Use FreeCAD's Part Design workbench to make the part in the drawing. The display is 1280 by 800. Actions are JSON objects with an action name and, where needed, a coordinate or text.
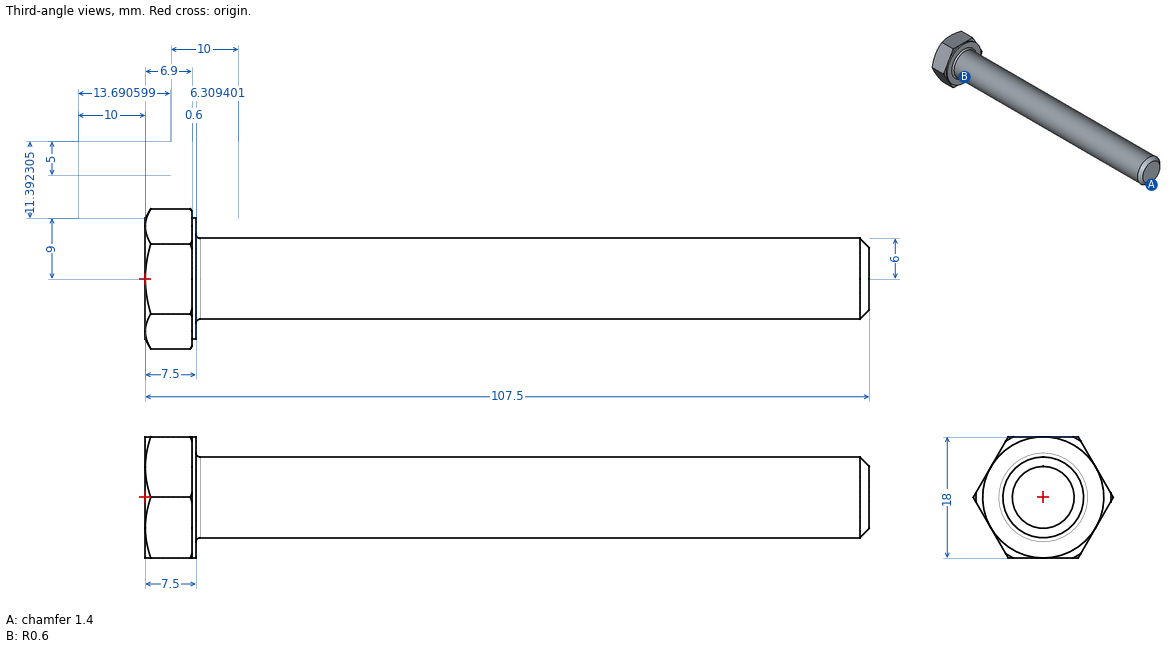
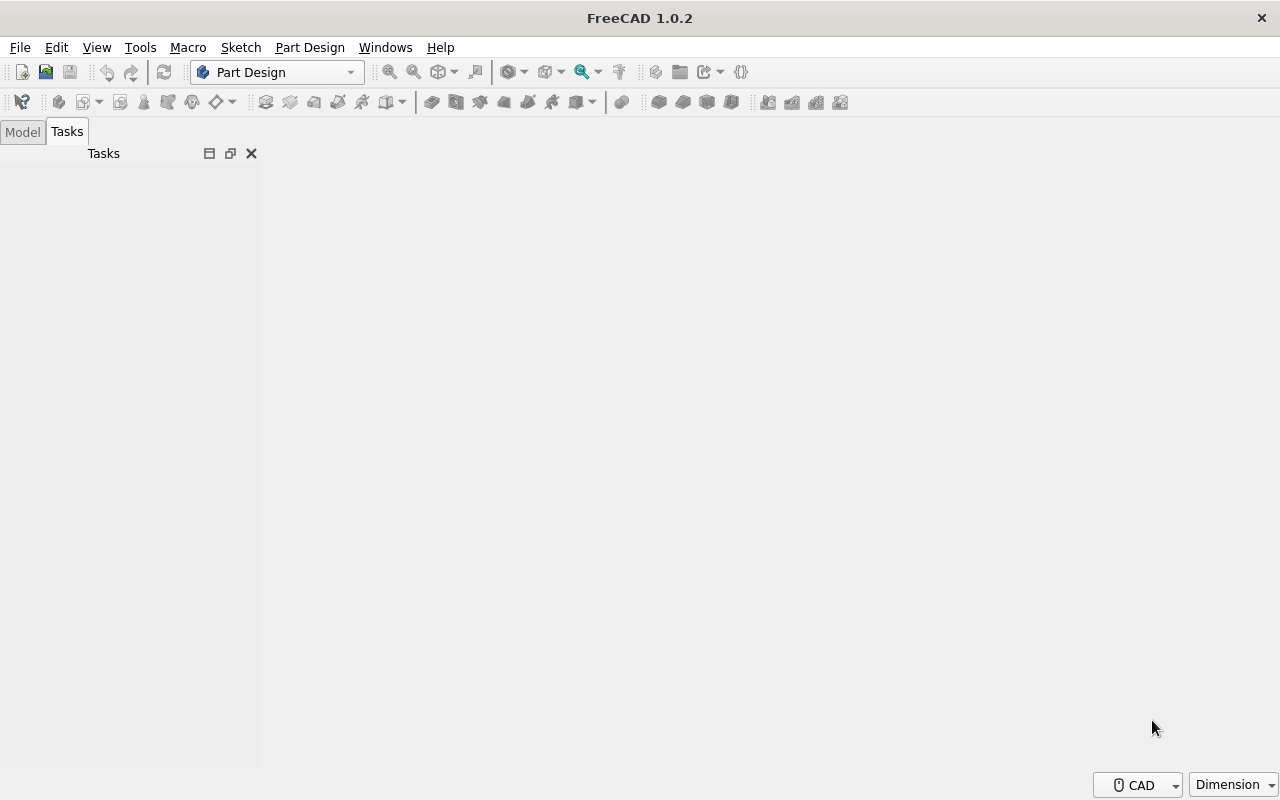
{"action": "key", "text": "ctrl+n"}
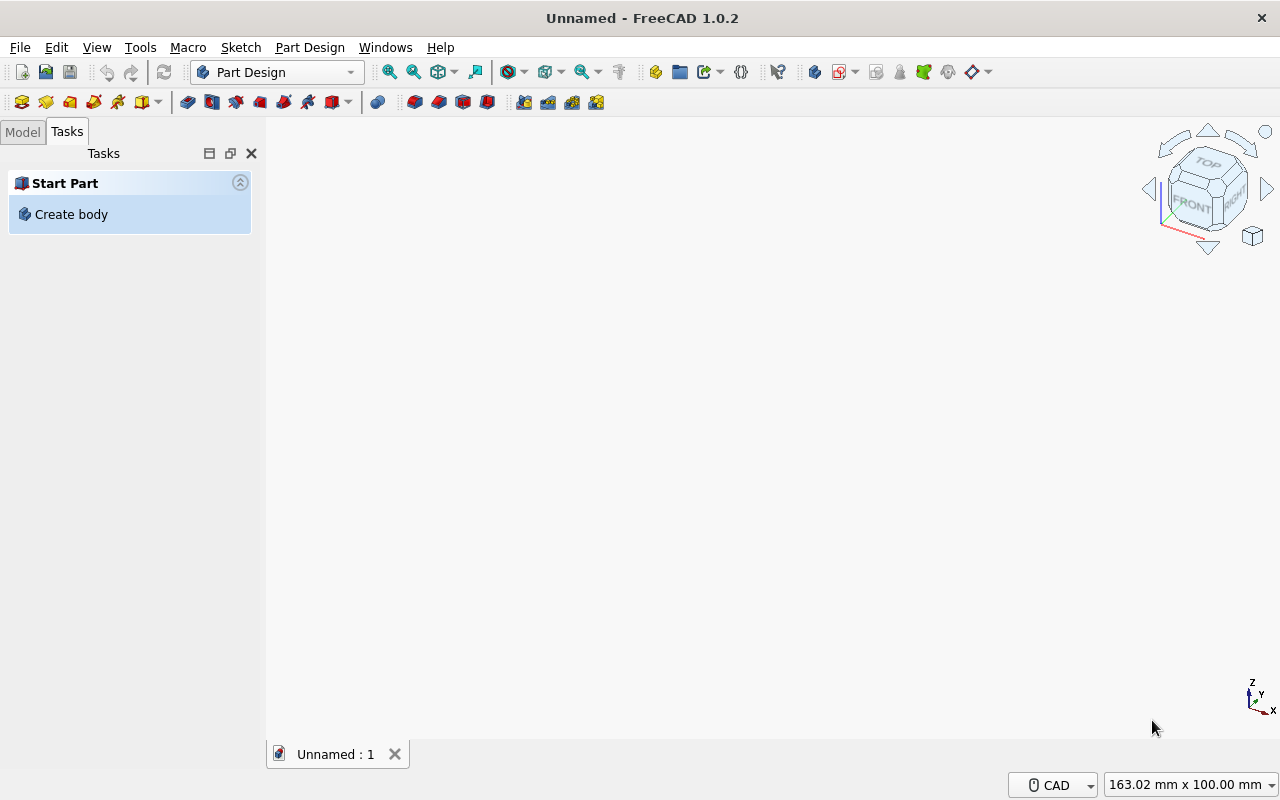
{"action": "left_click", "coordinate": [840, 72]}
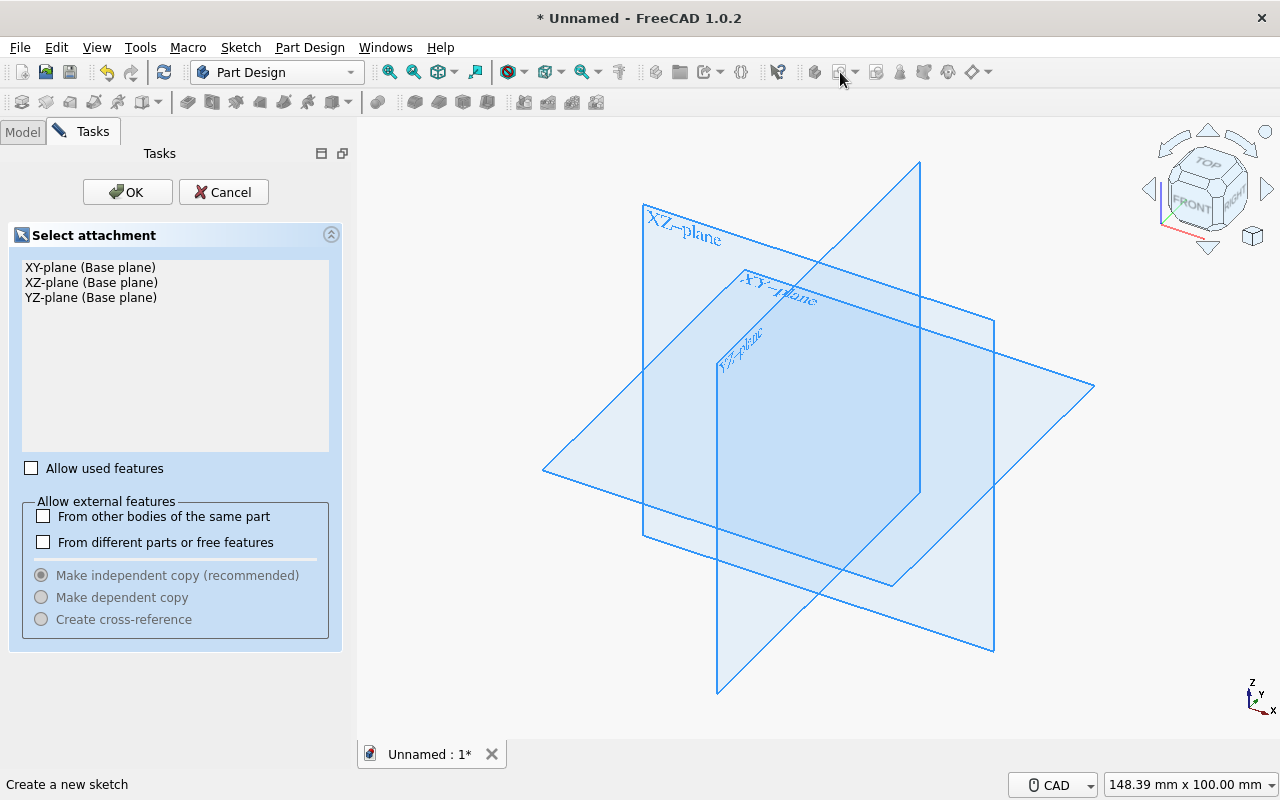
{"action": "left_click", "coordinate": [82, 298]}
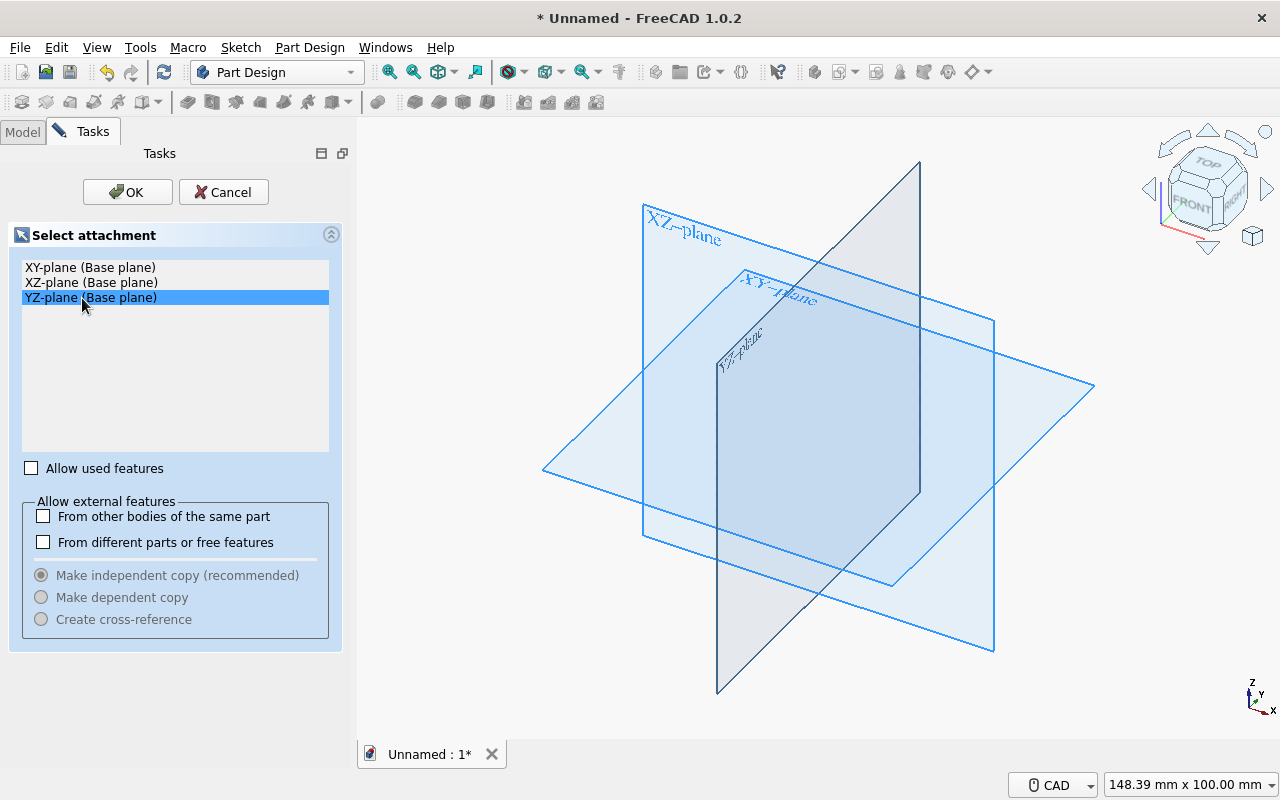
{"action": "left_click", "coordinate": [128, 192]}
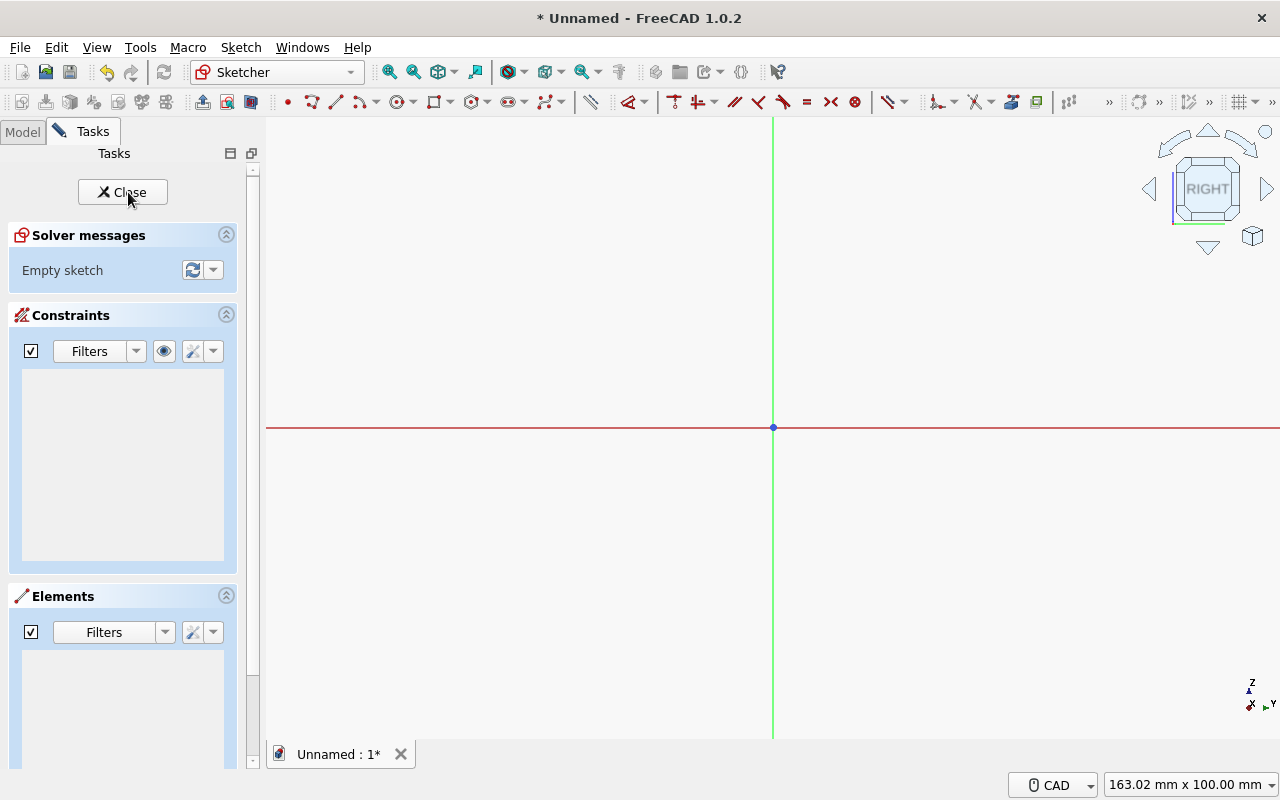
{"action": "scroll", "coordinate": [803, 428], "scroll_direction": "up", "scroll_amount": 6}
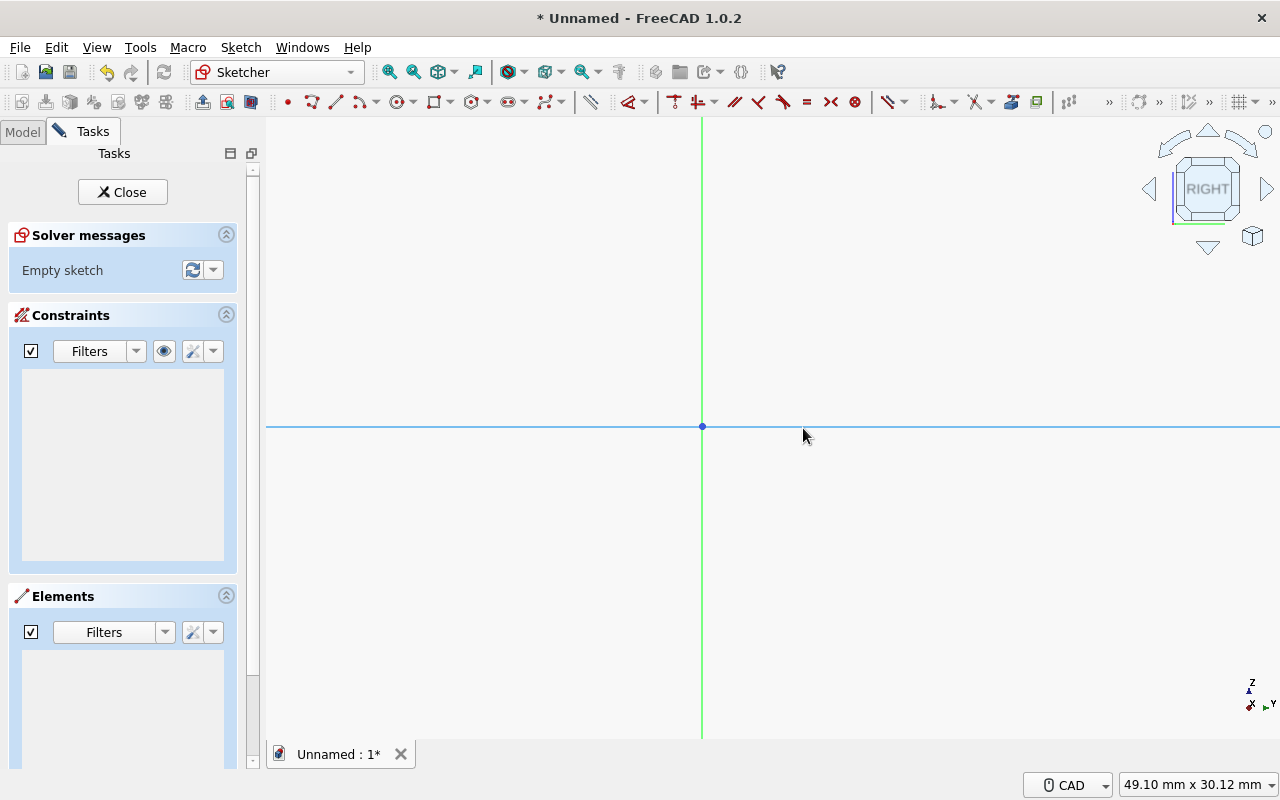
{"action": "left_click", "coordinate": [472, 102]}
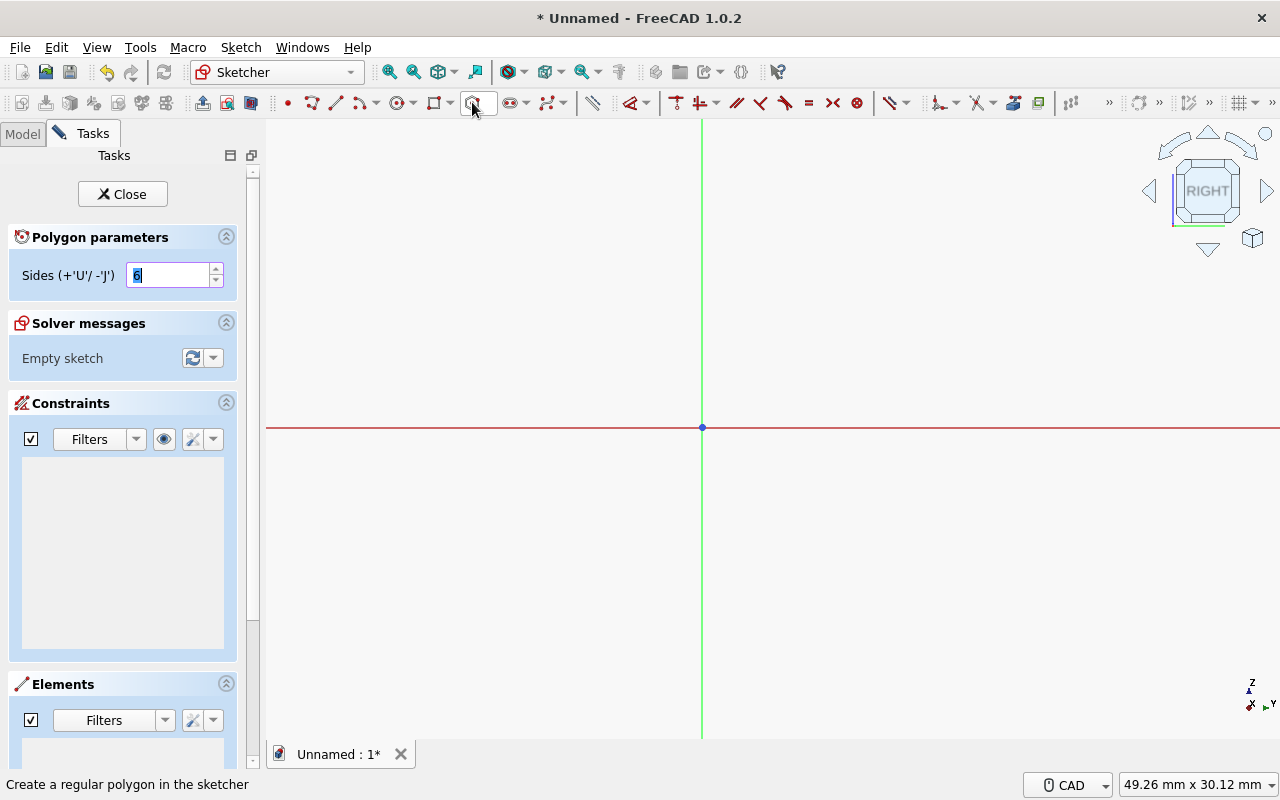
{"action": "left_click", "coordinate": [702, 428]}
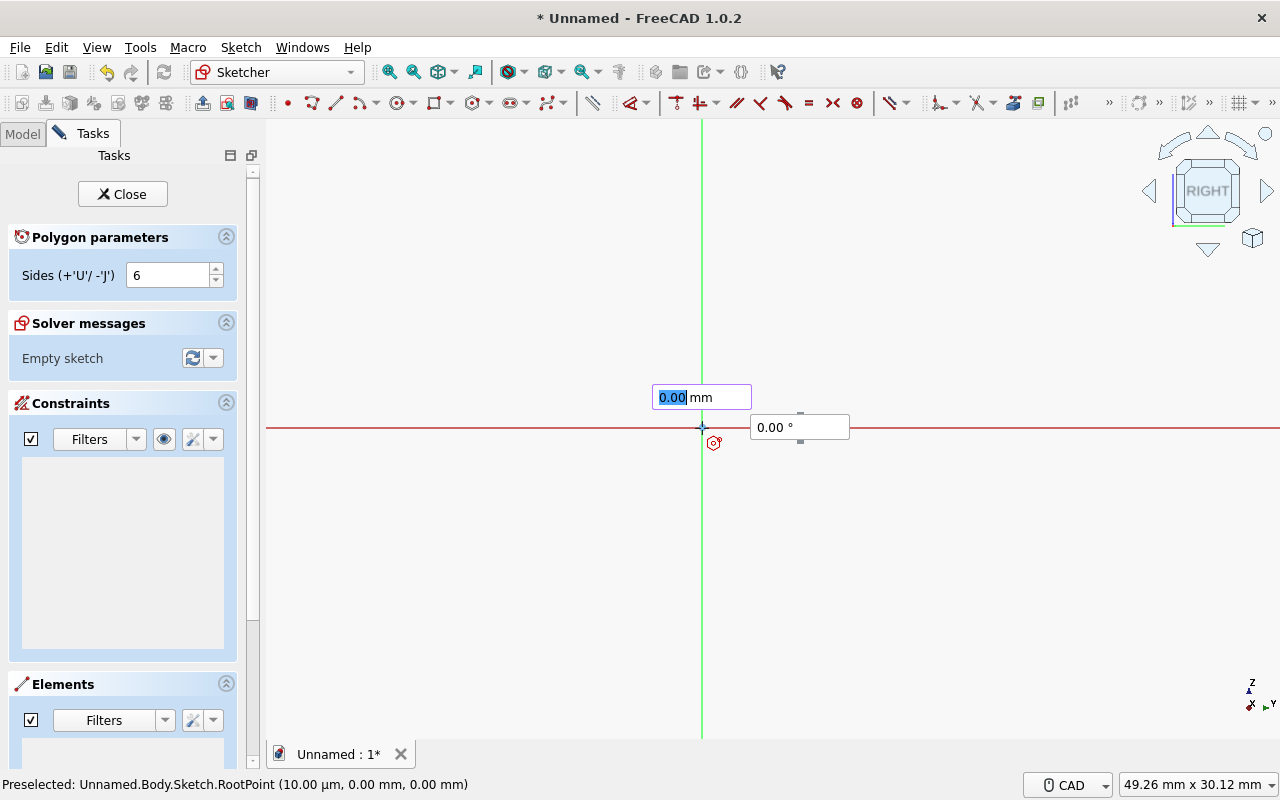
{"action": "left_click", "coordinate": [916, 428]}
{"action": "right_click", "coordinate": [916, 428]}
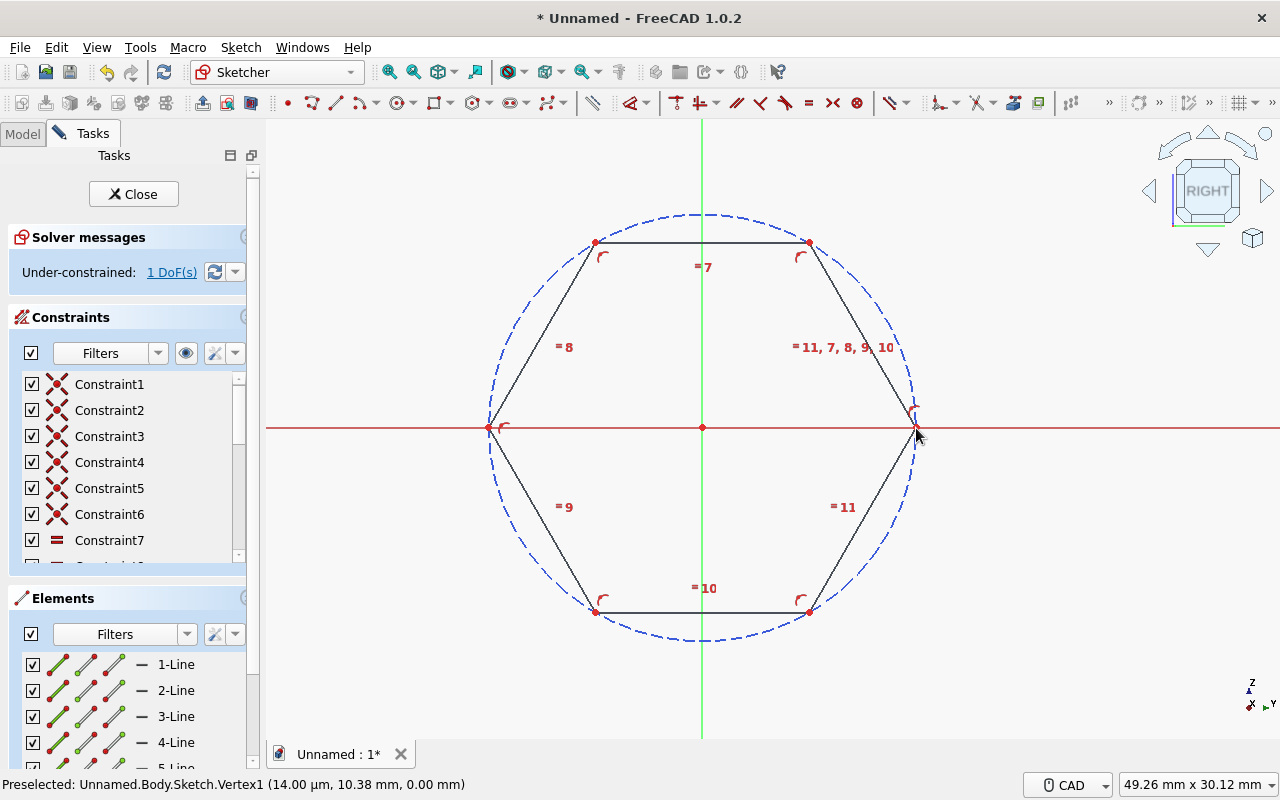
{"action": "key", "text": "d"}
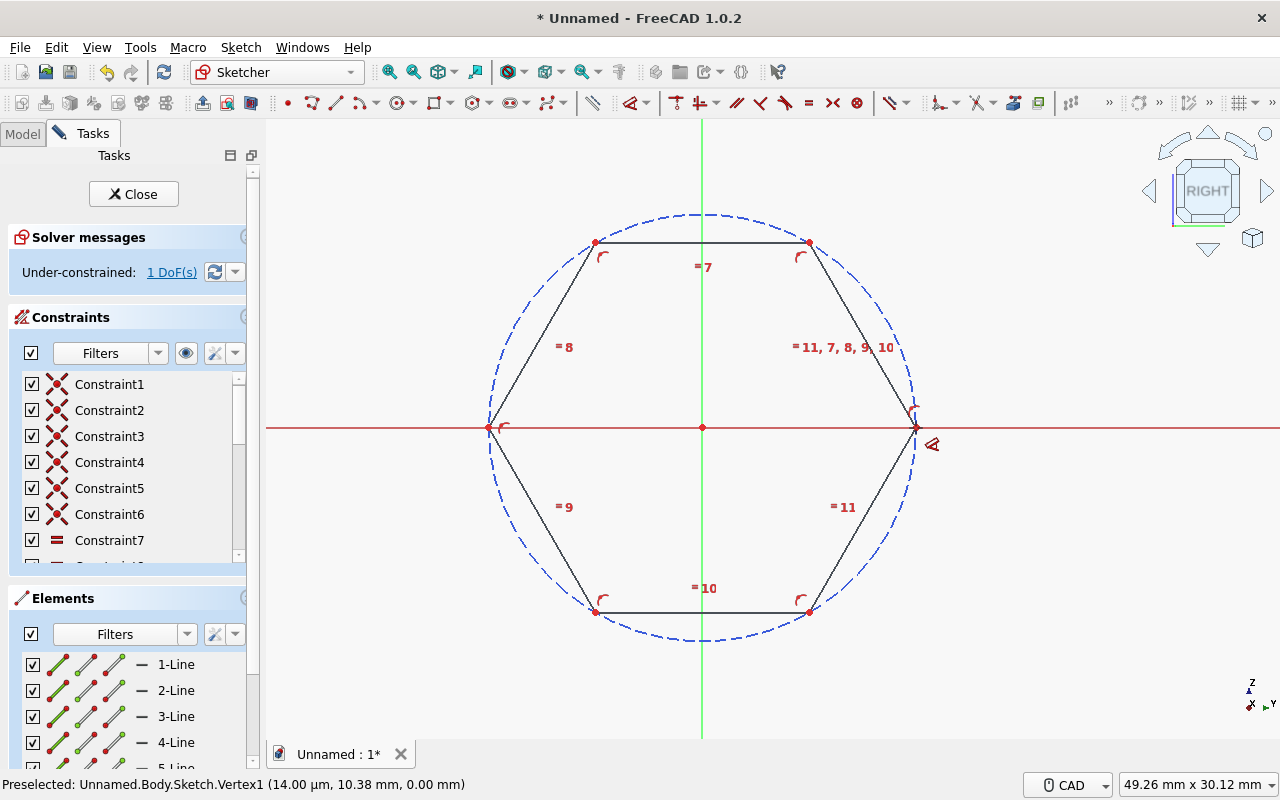
{"action": "left_click", "coordinate": [596, 613]}